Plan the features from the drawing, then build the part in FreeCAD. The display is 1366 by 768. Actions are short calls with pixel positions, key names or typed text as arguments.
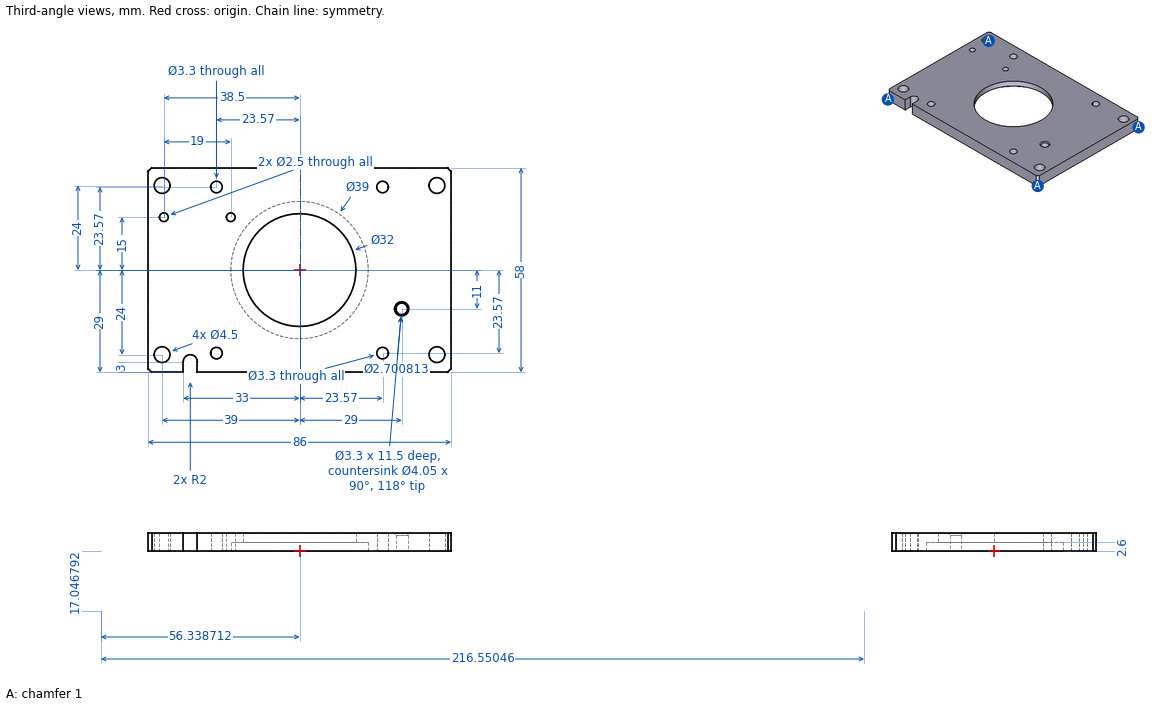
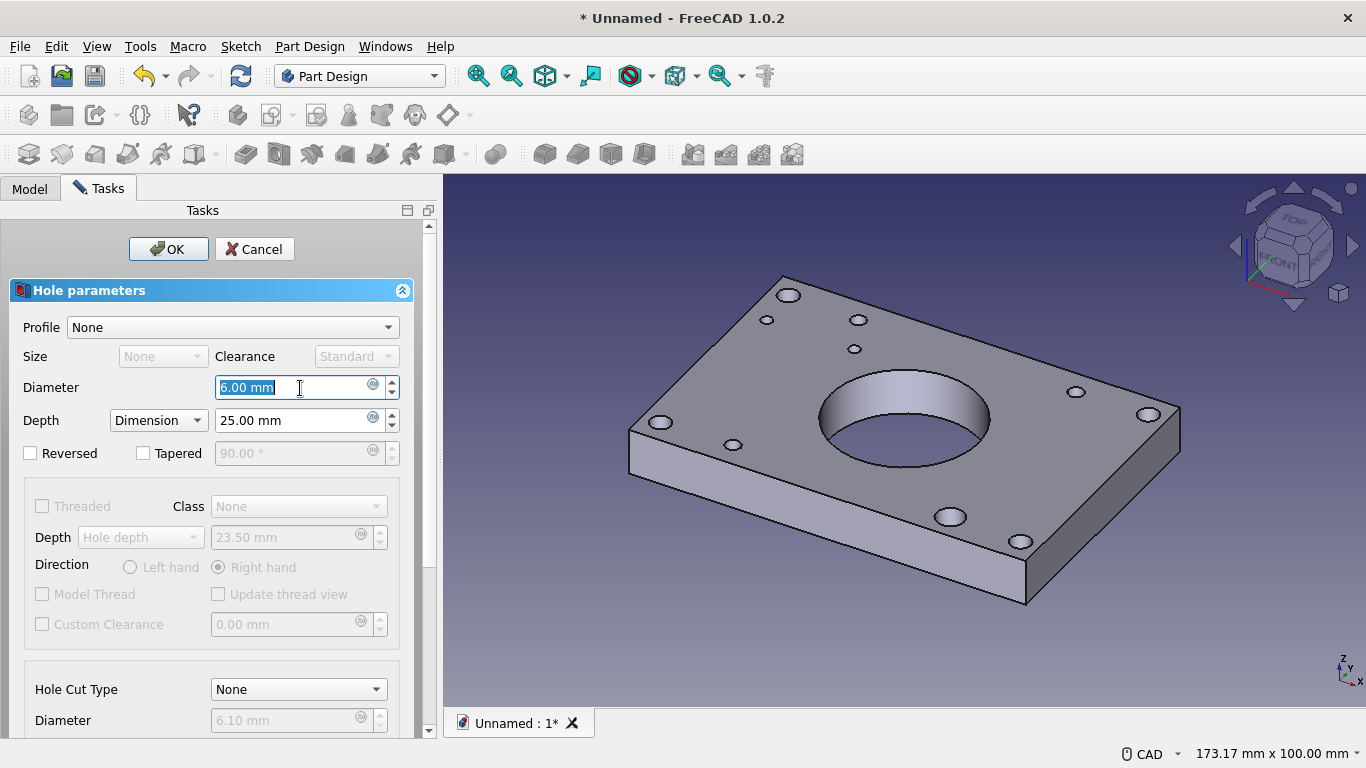
text(3.3)
key(Tab)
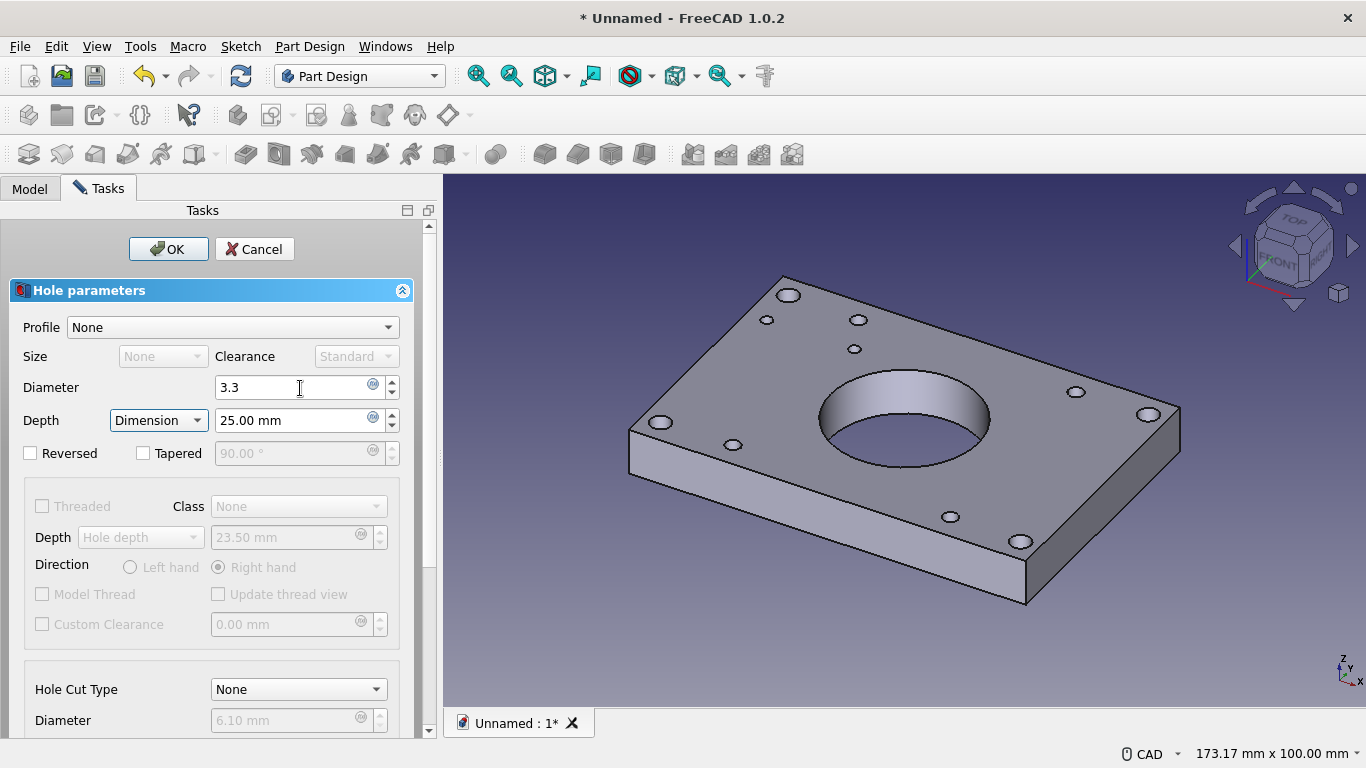
click(160, 420)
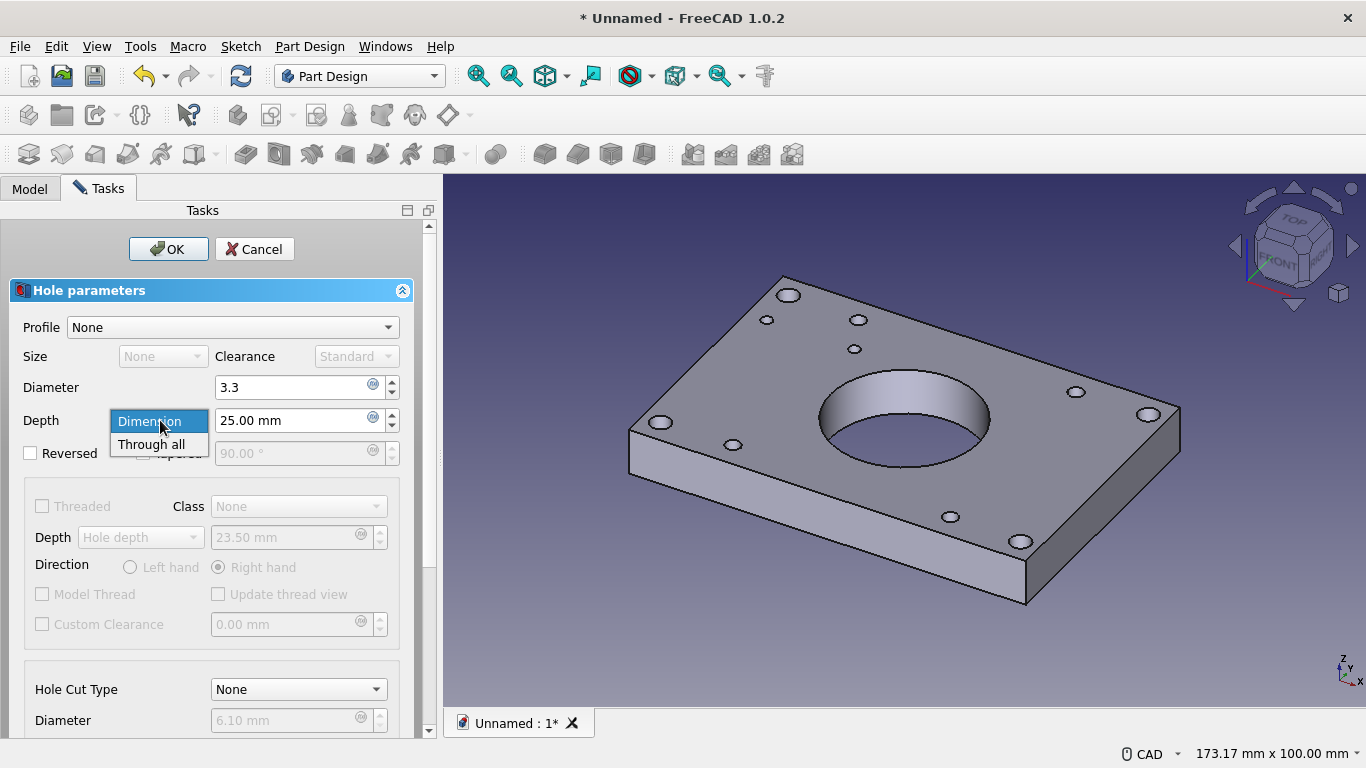
click(158, 444)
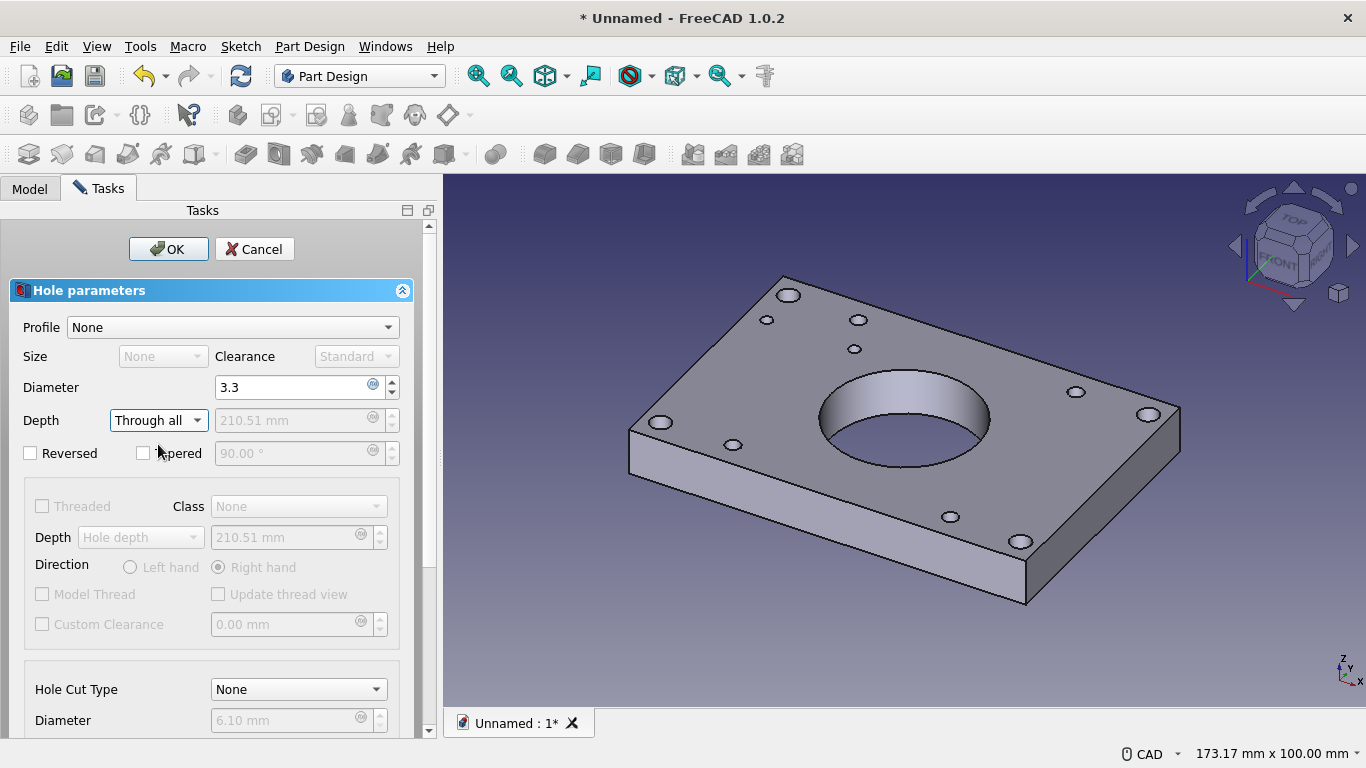
click(169, 249)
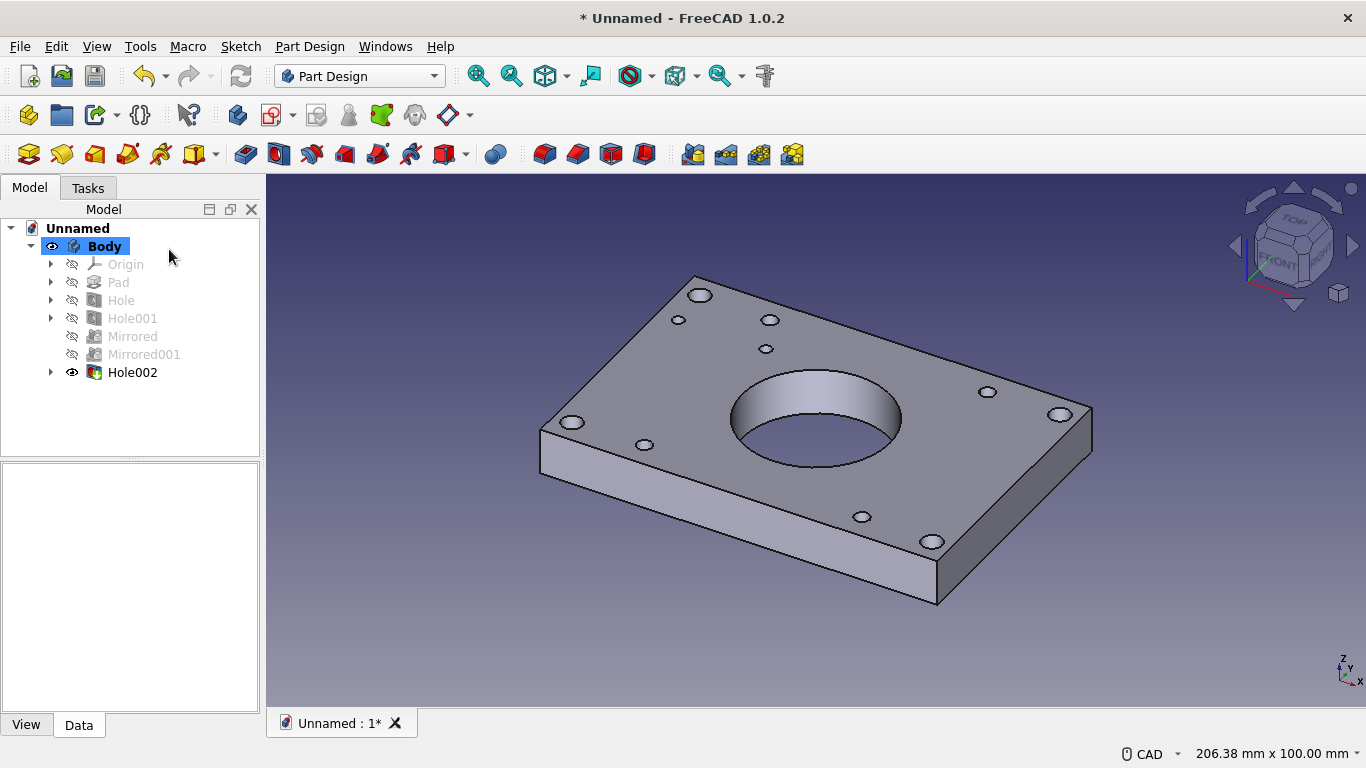
click(680, 402)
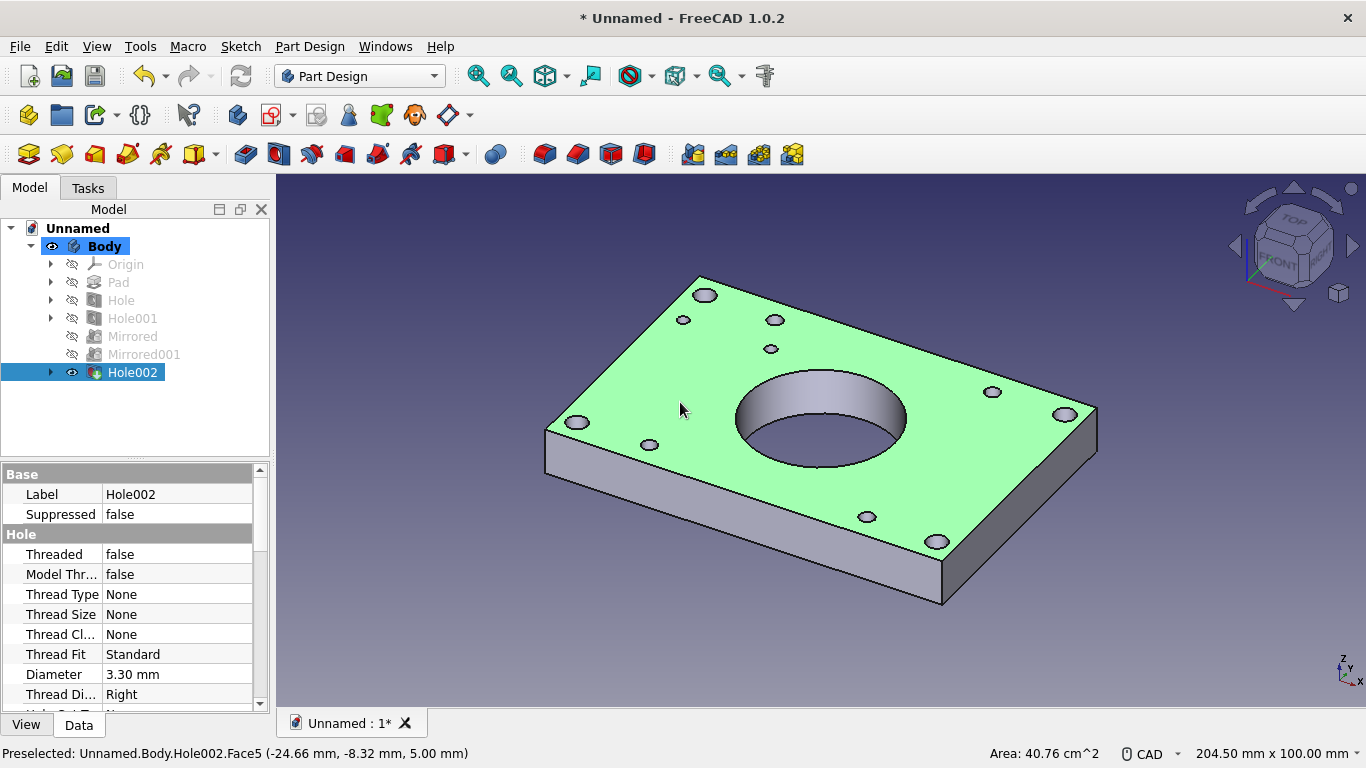
click(270, 116)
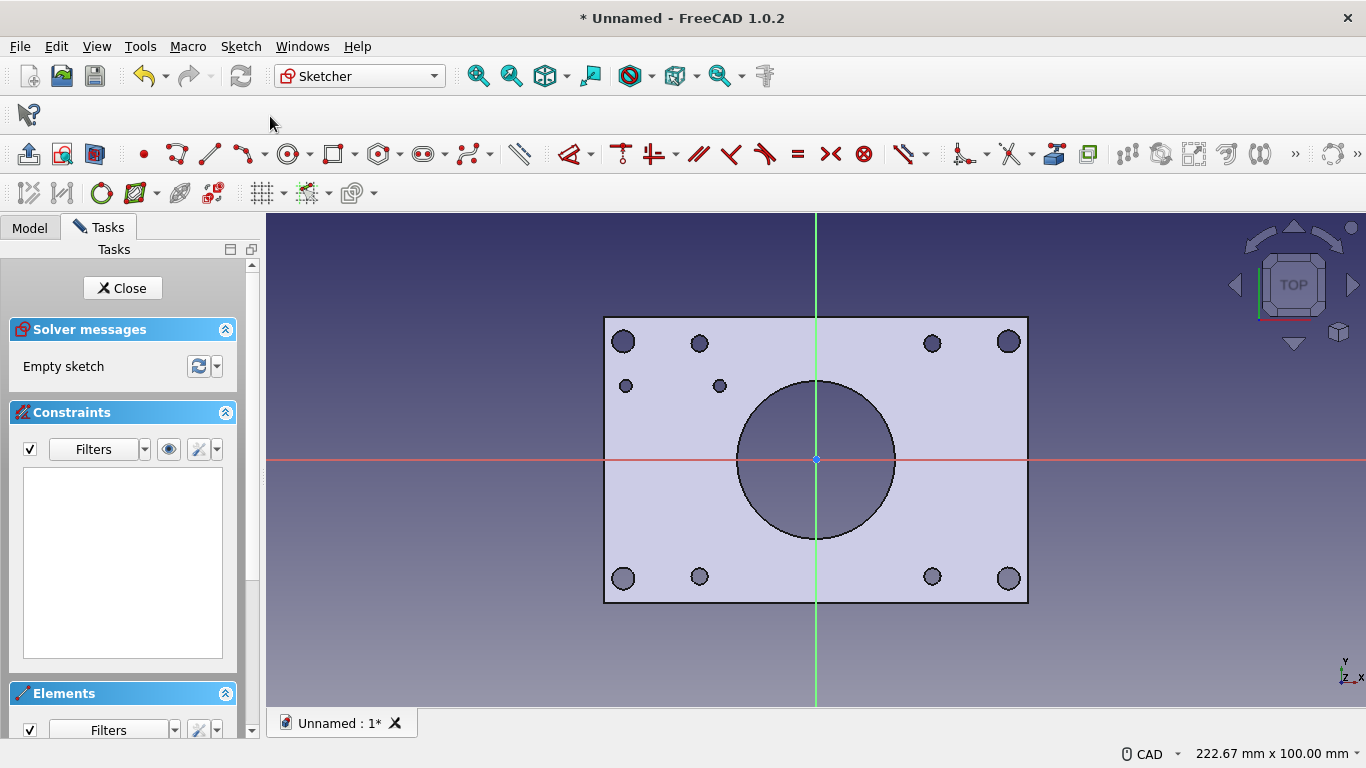
scroll(652, 613, up, 11)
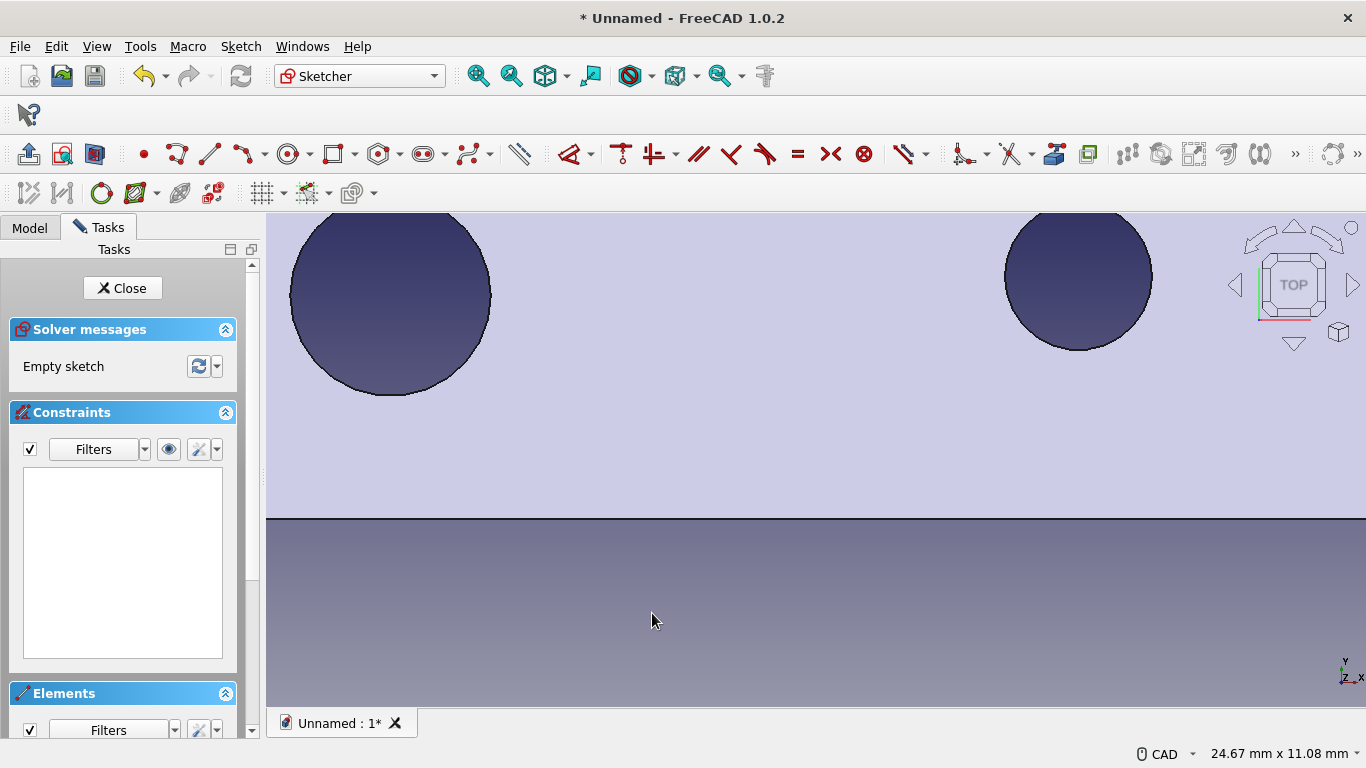
key(g)
key(s)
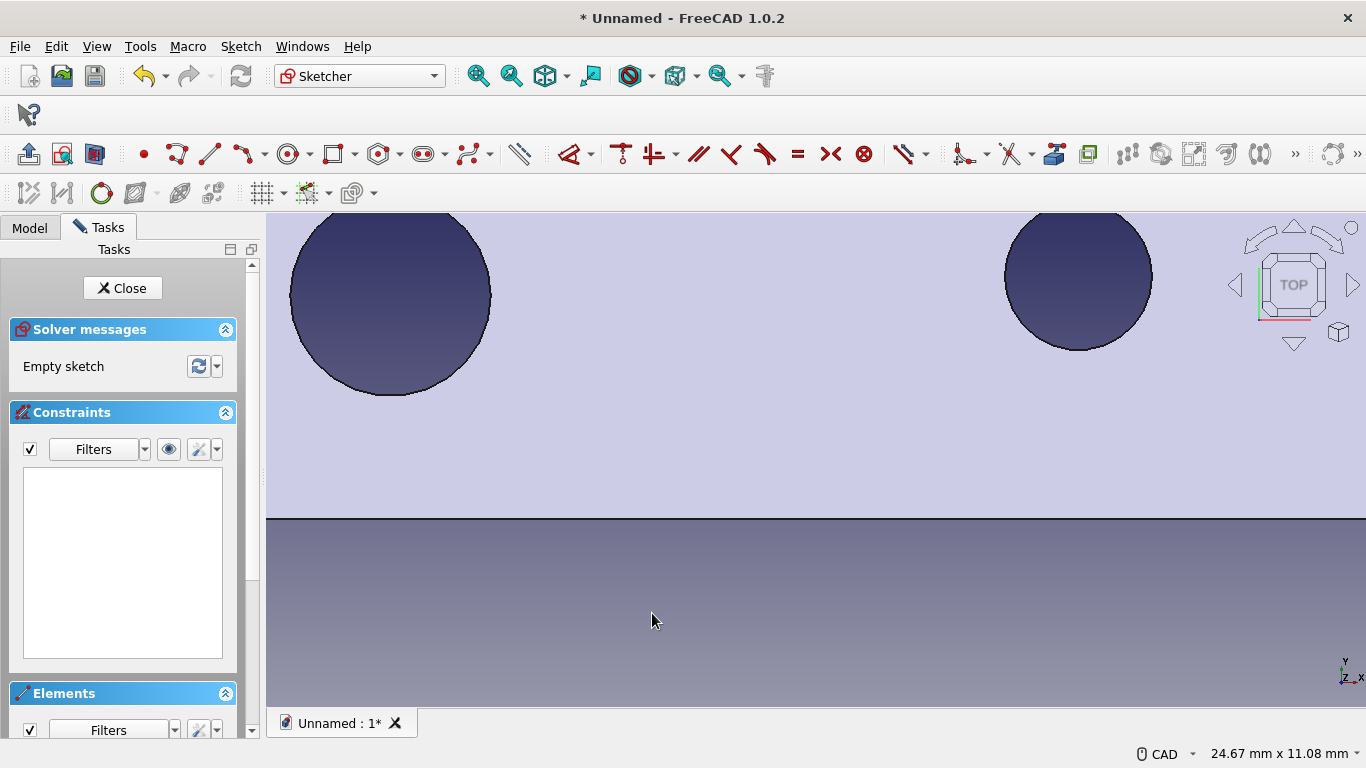
click(747, 519)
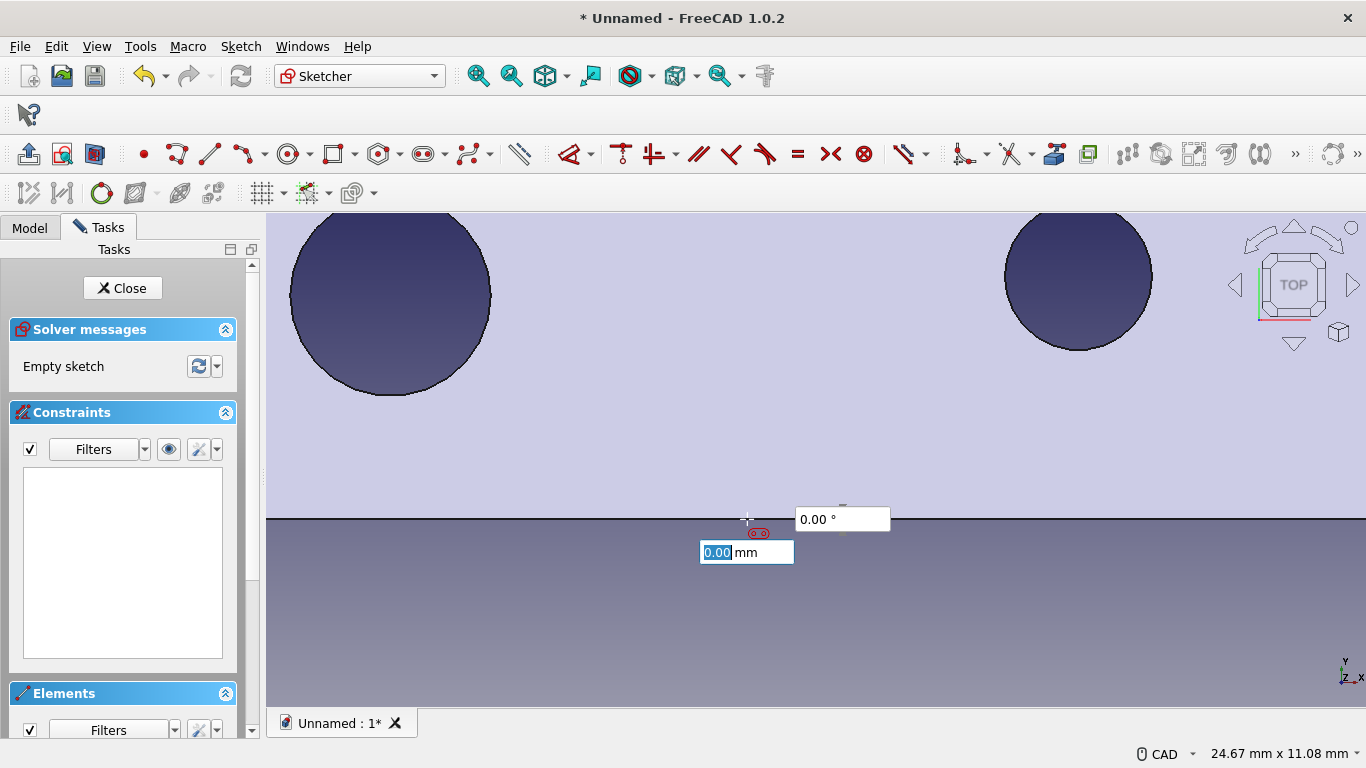
click(747, 385)